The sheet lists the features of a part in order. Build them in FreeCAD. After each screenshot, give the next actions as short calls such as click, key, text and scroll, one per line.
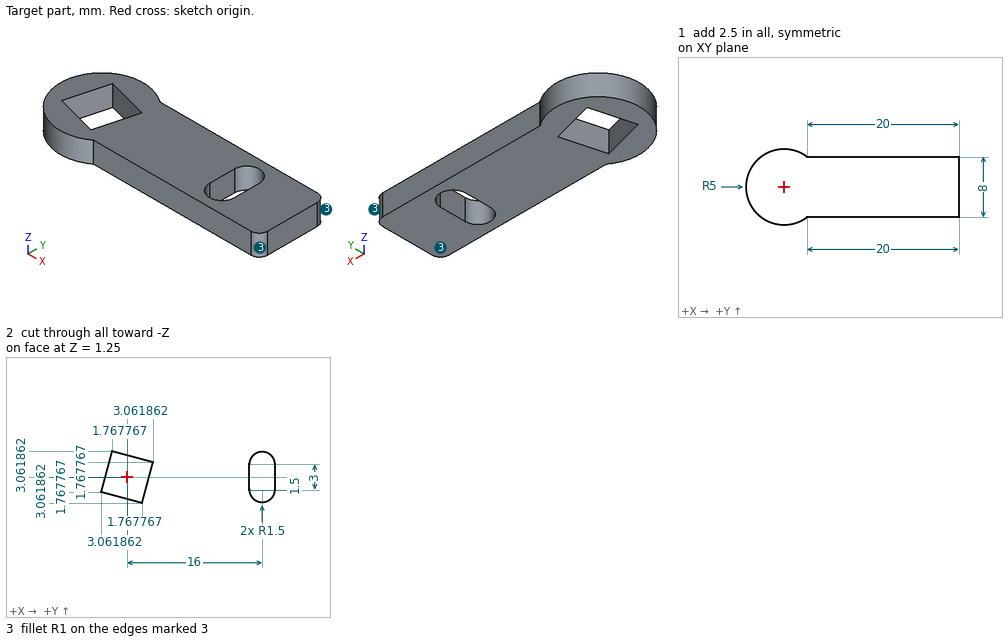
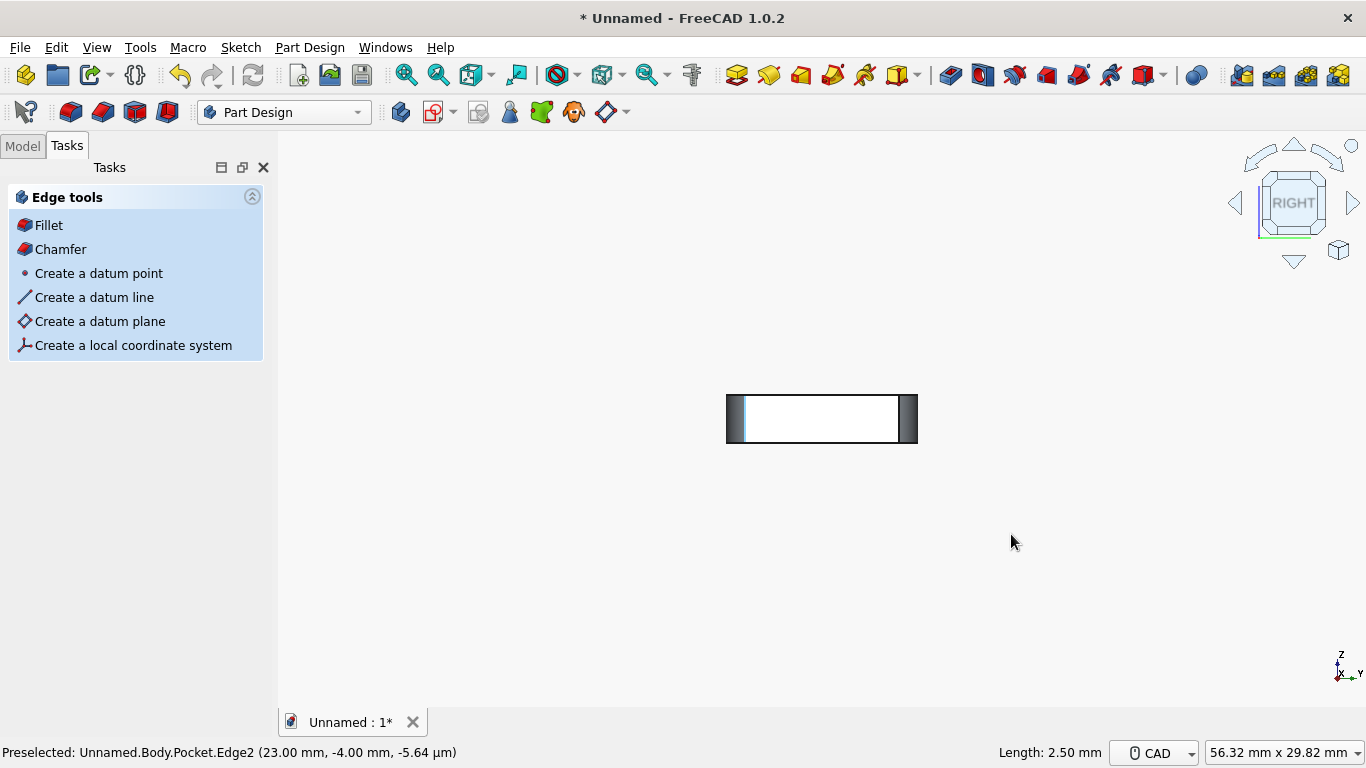
click(408, 76)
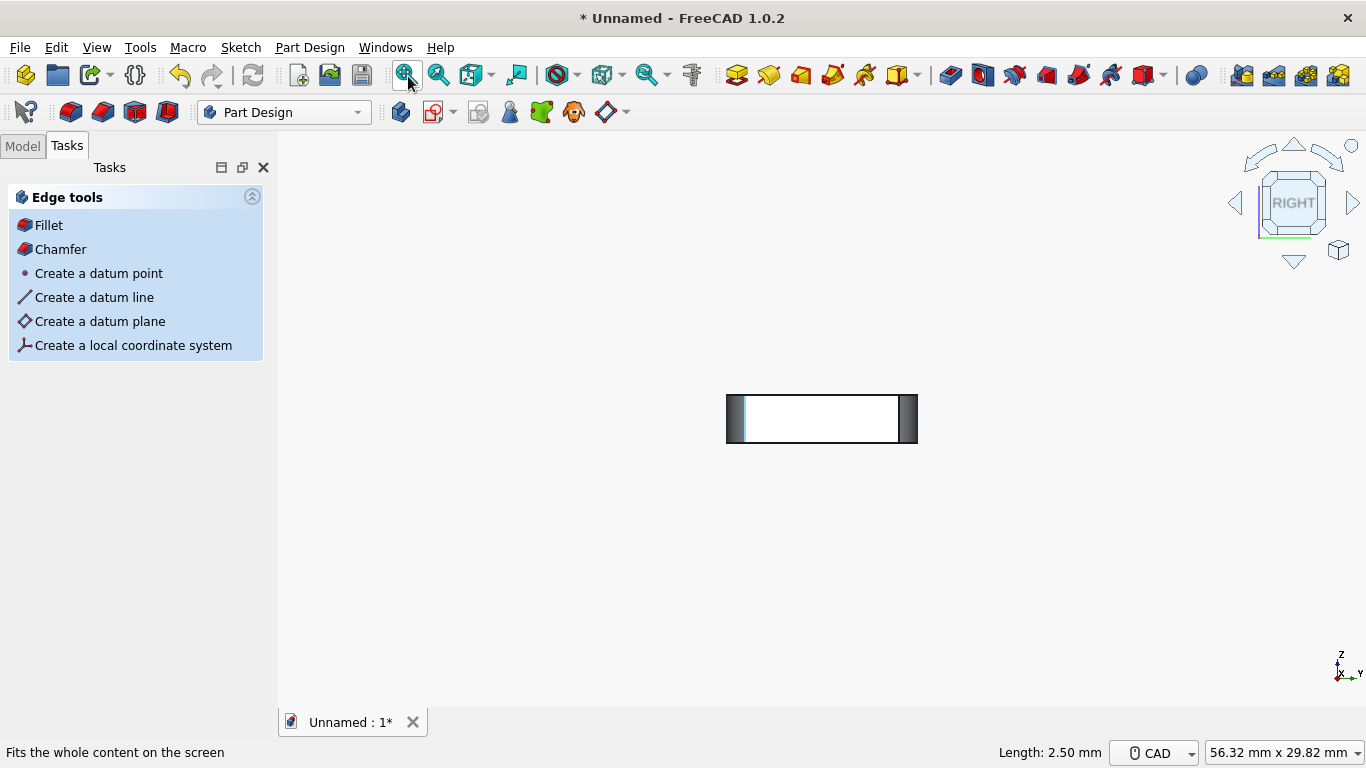
click(899, 418, ctrl)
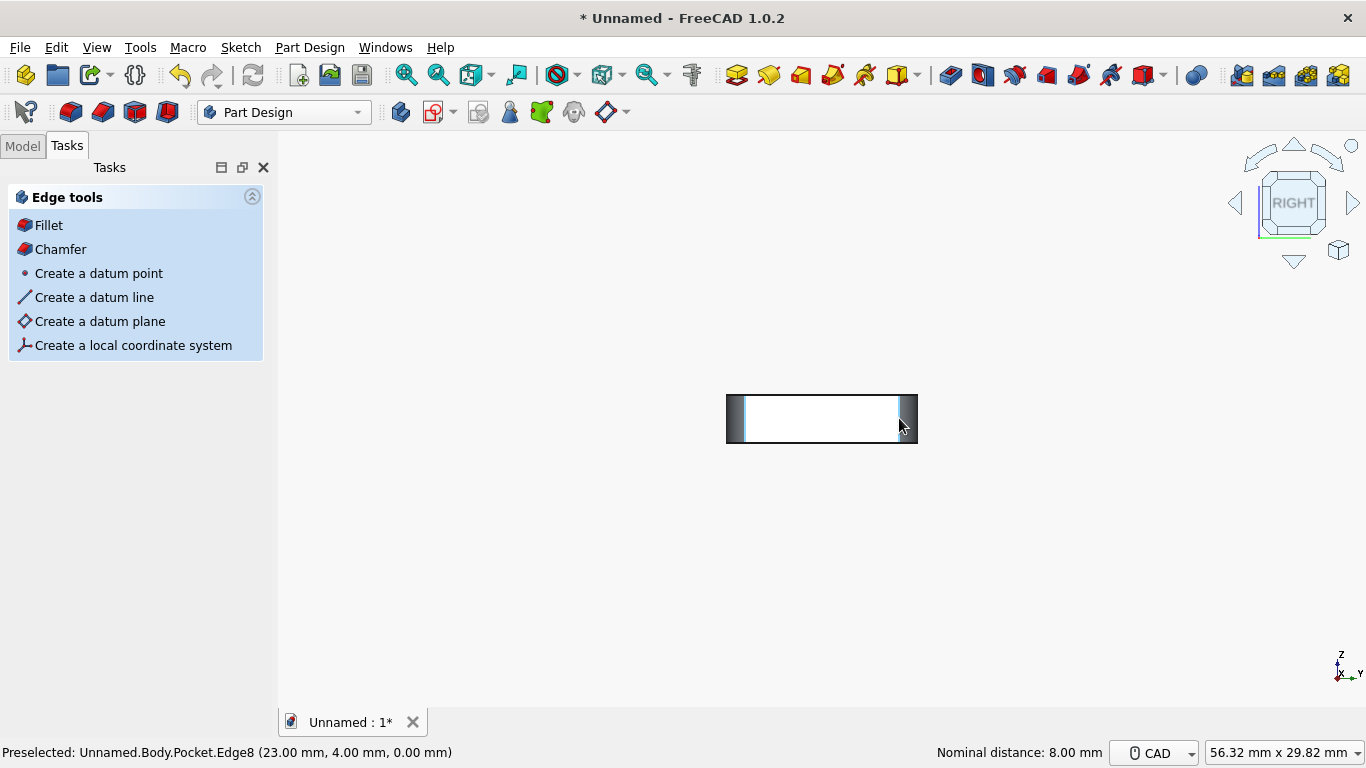
click(72, 112)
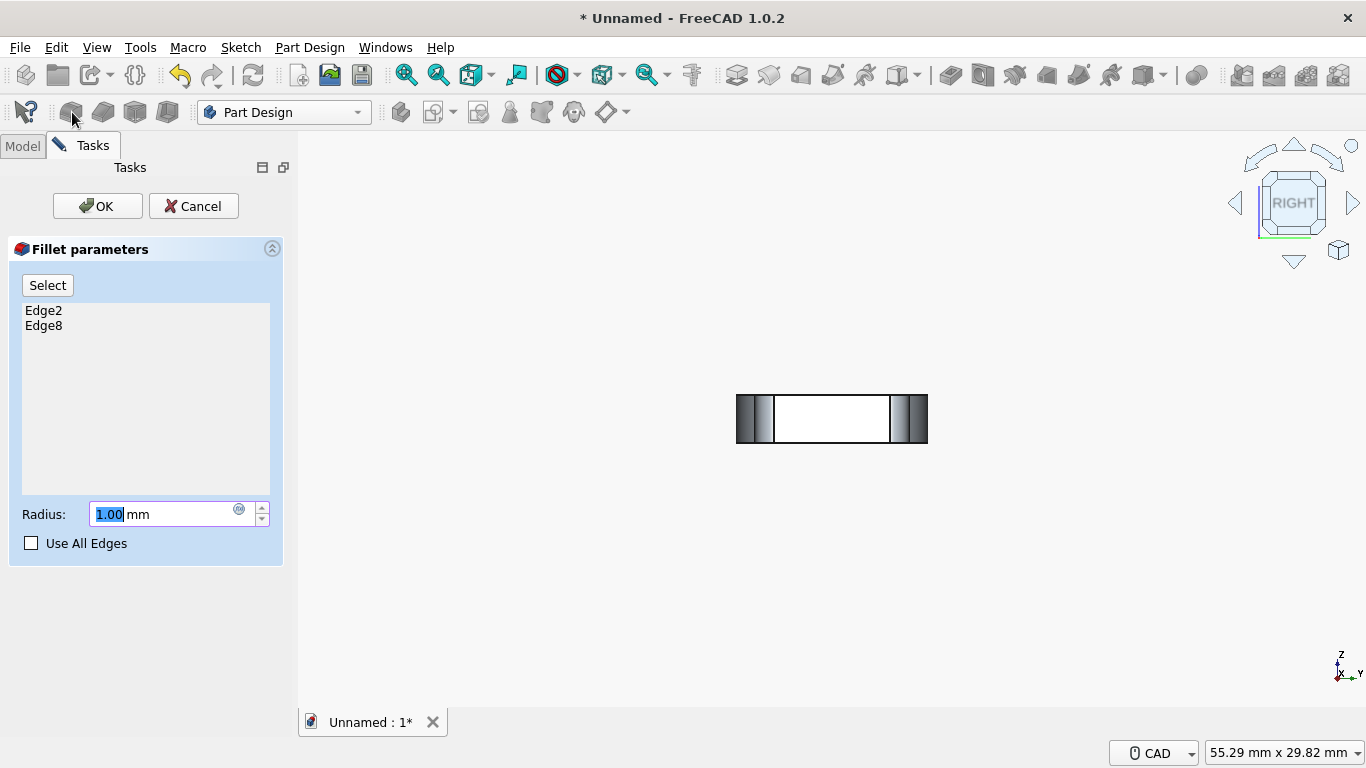
text(1)
key(Tab)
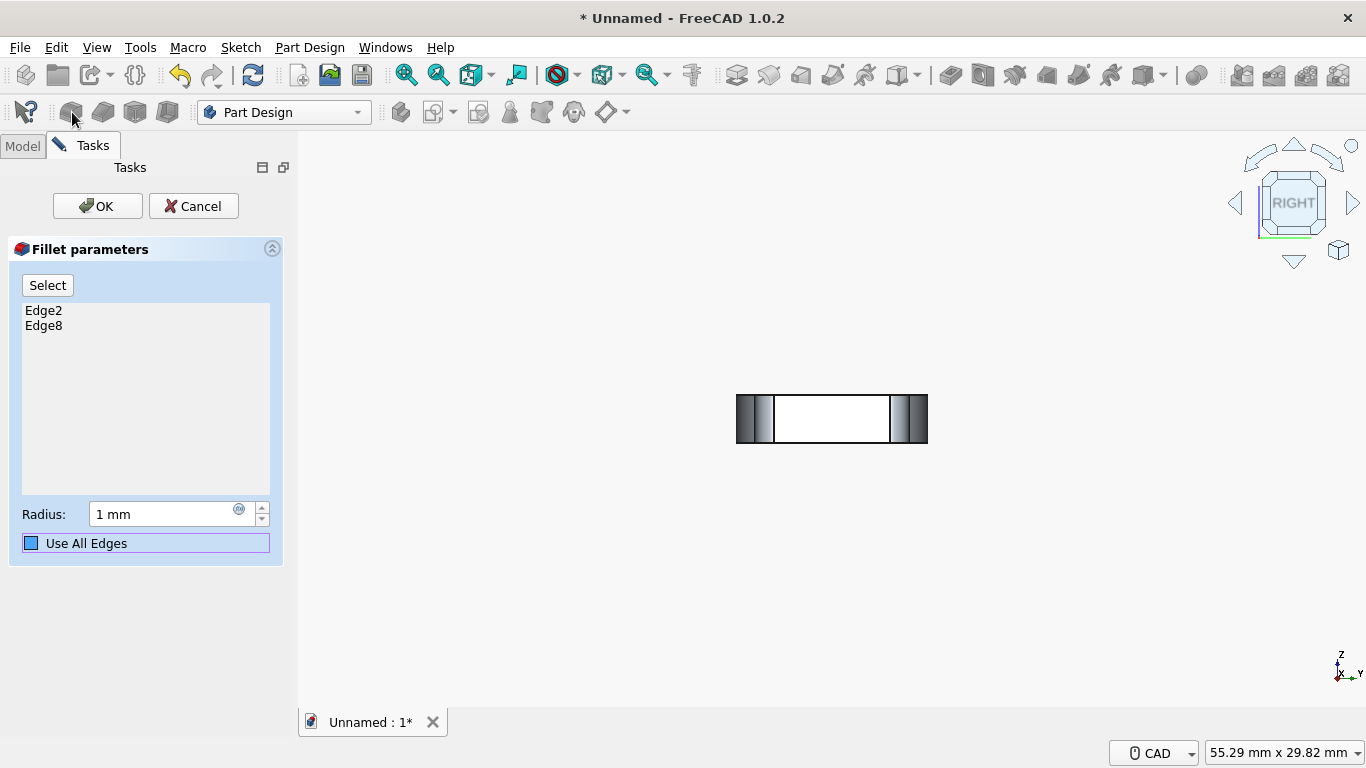
click(98, 206)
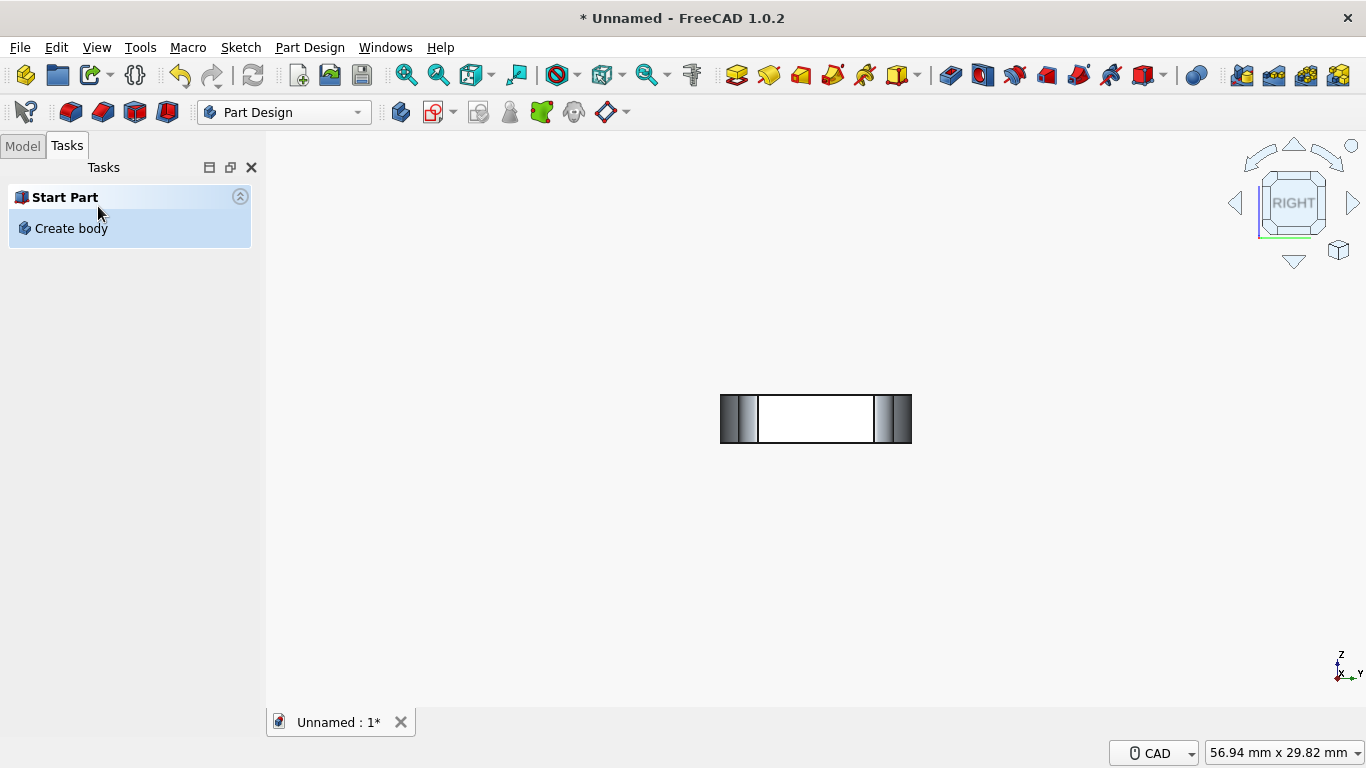
key(0)